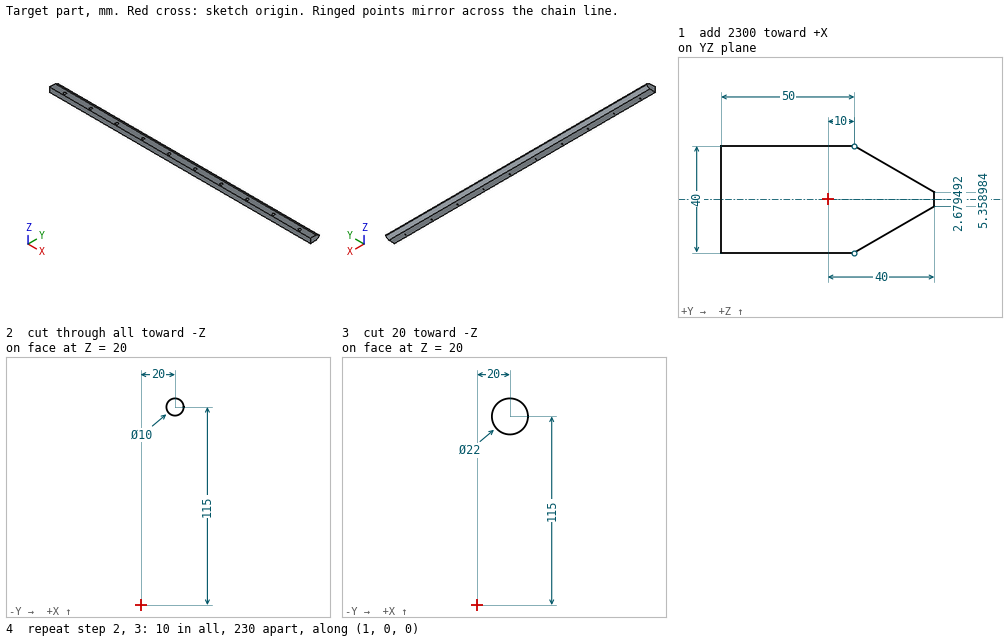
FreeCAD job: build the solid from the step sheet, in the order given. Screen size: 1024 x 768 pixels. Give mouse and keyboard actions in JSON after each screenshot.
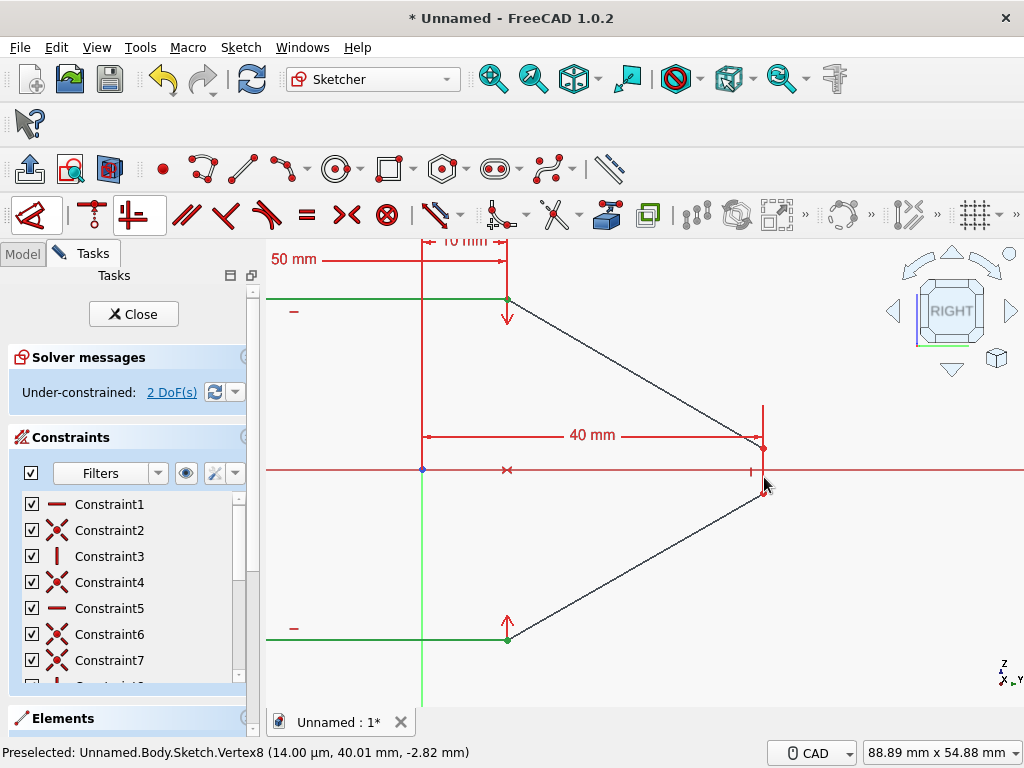
{"action": "left_click", "coordinate": [763, 476]}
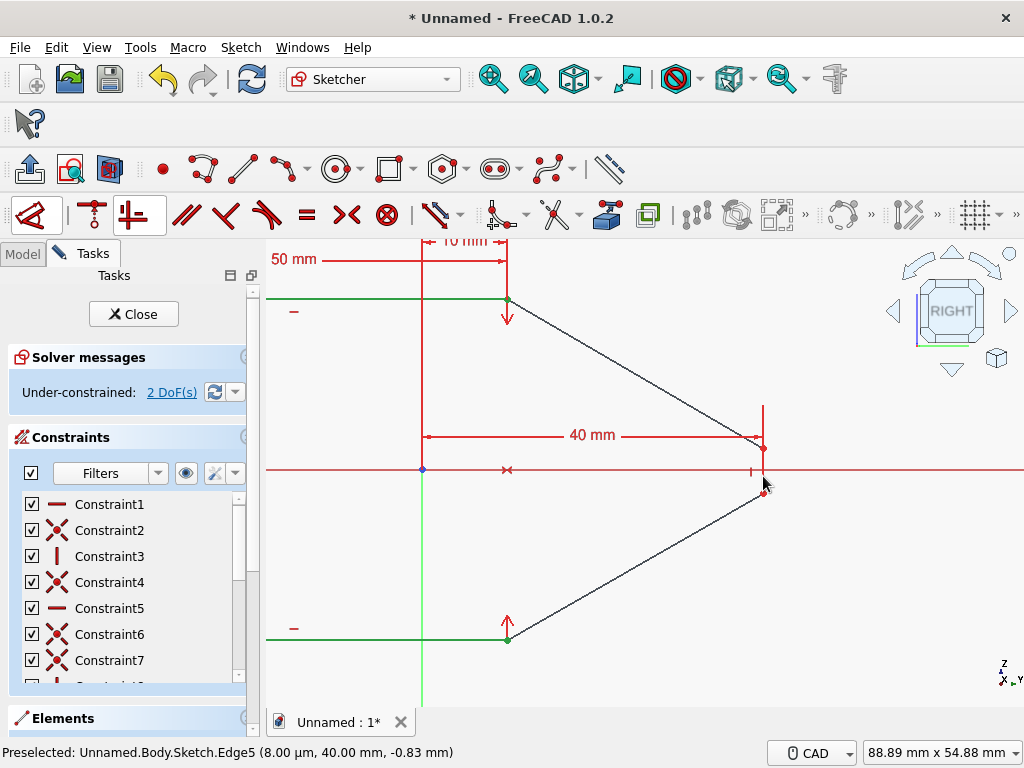
{"action": "key", "text": "i"}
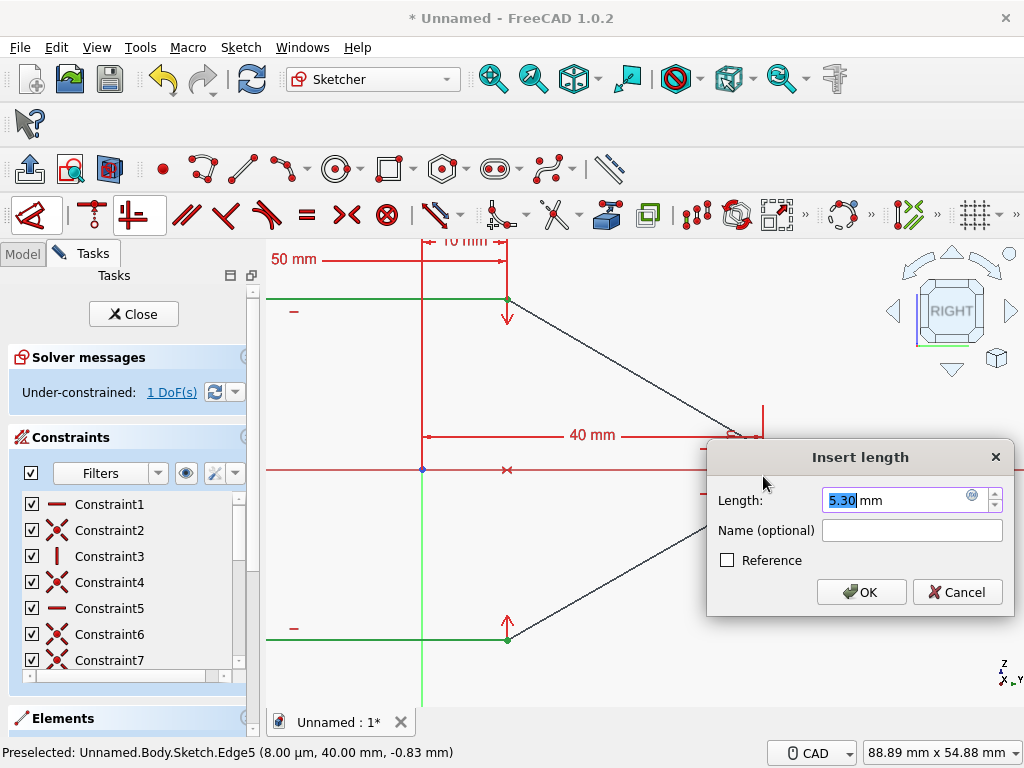
{"action": "type", "text": "5.358984"}
{"action": "key", "text": "Return"}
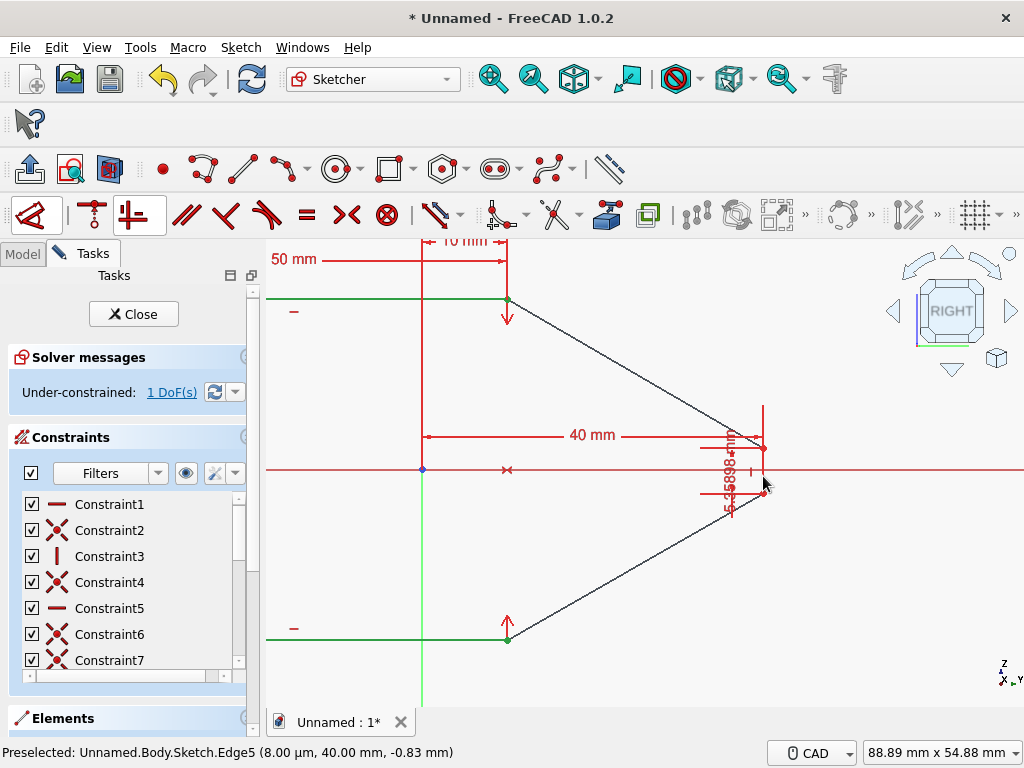
{"action": "scroll", "coordinate": [763, 494], "scroll_direction": "up", "scroll_amount": 3}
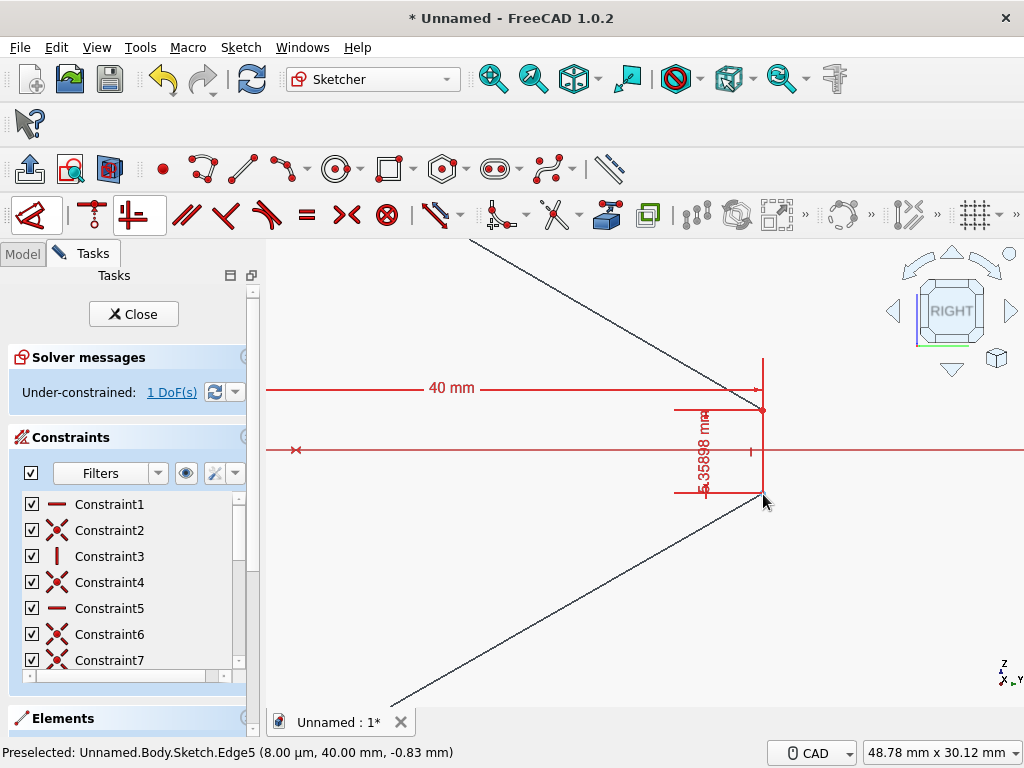
{"action": "left_click", "coordinate": [763, 493]}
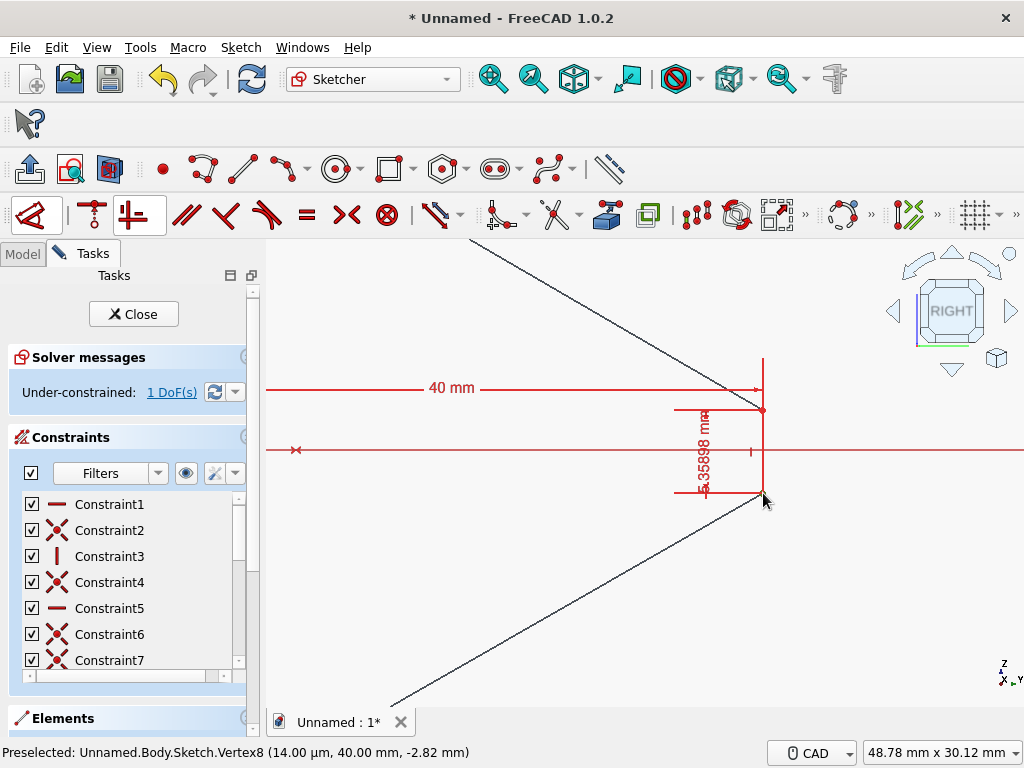
{"action": "key", "text": "i"}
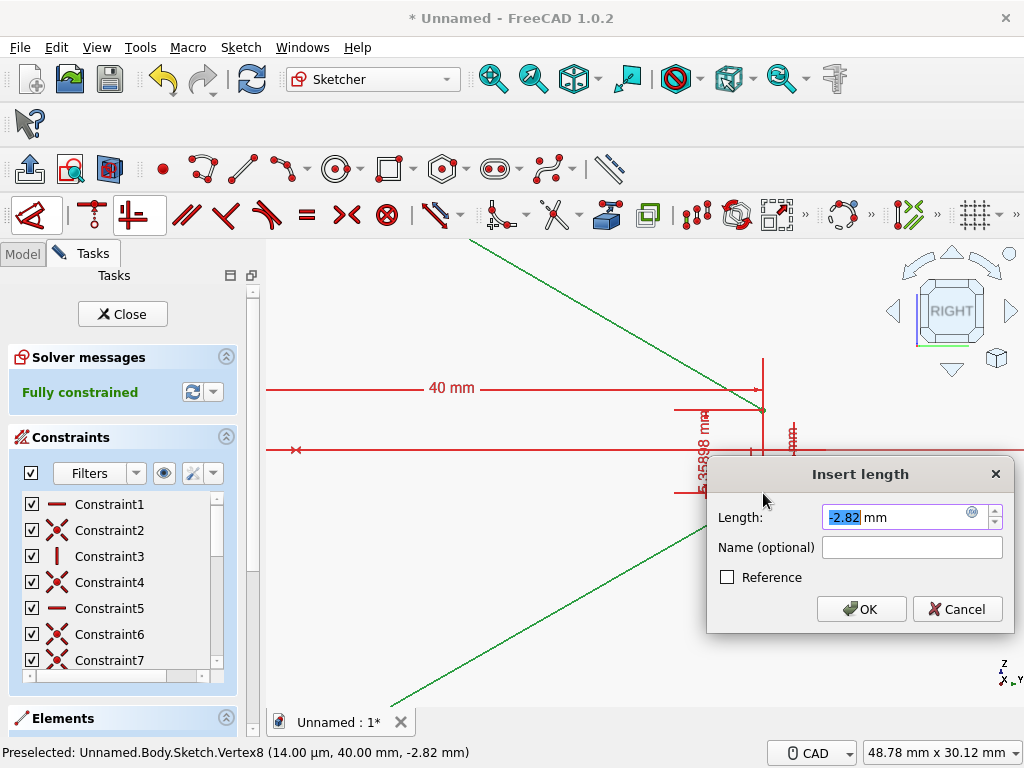
{"action": "type", "text": "-2.679492"}
{"action": "key", "text": "Return"}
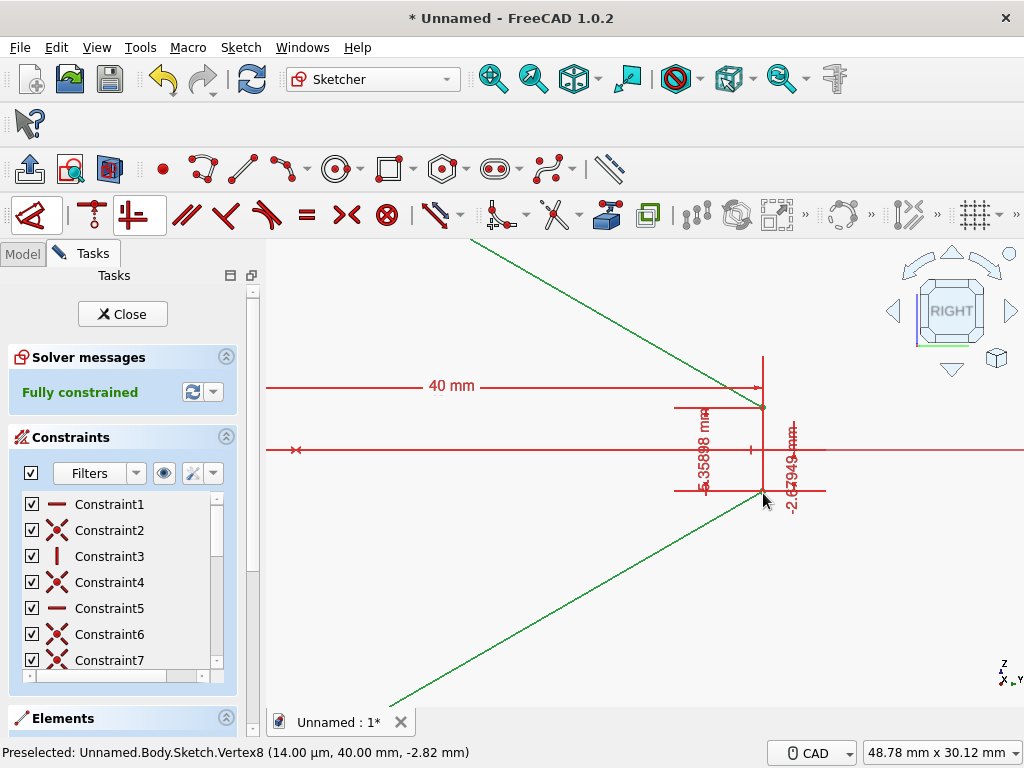
{"action": "left_click", "coordinate": [123, 314]}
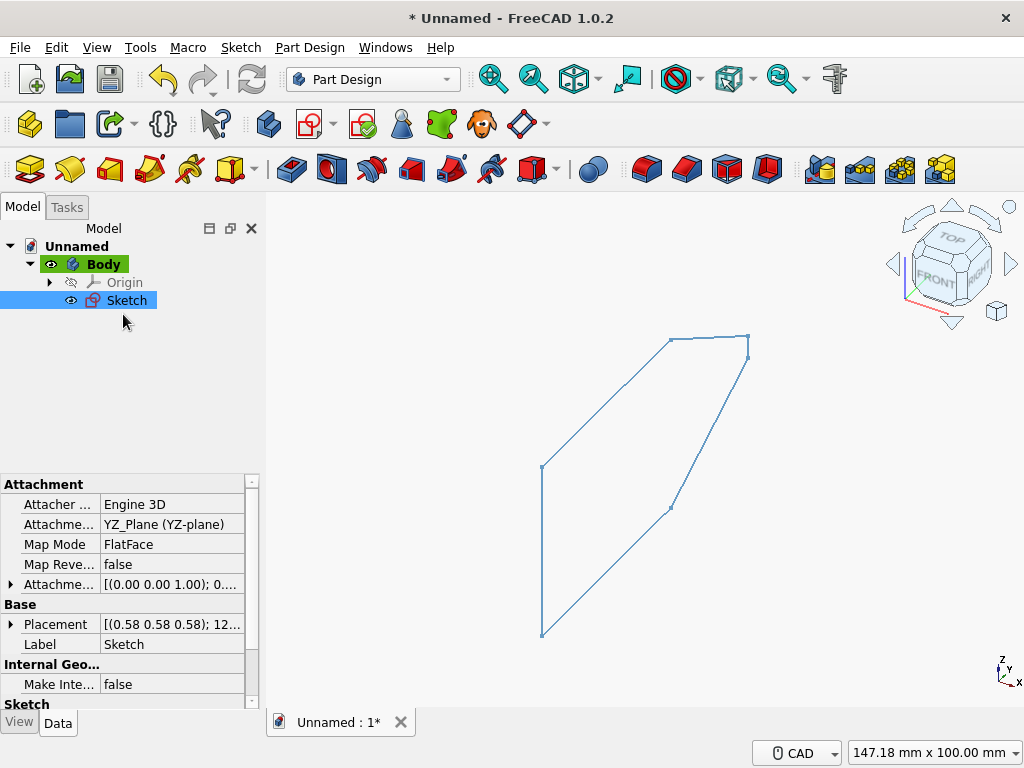
{"action": "left_click", "coordinate": [30, 170]}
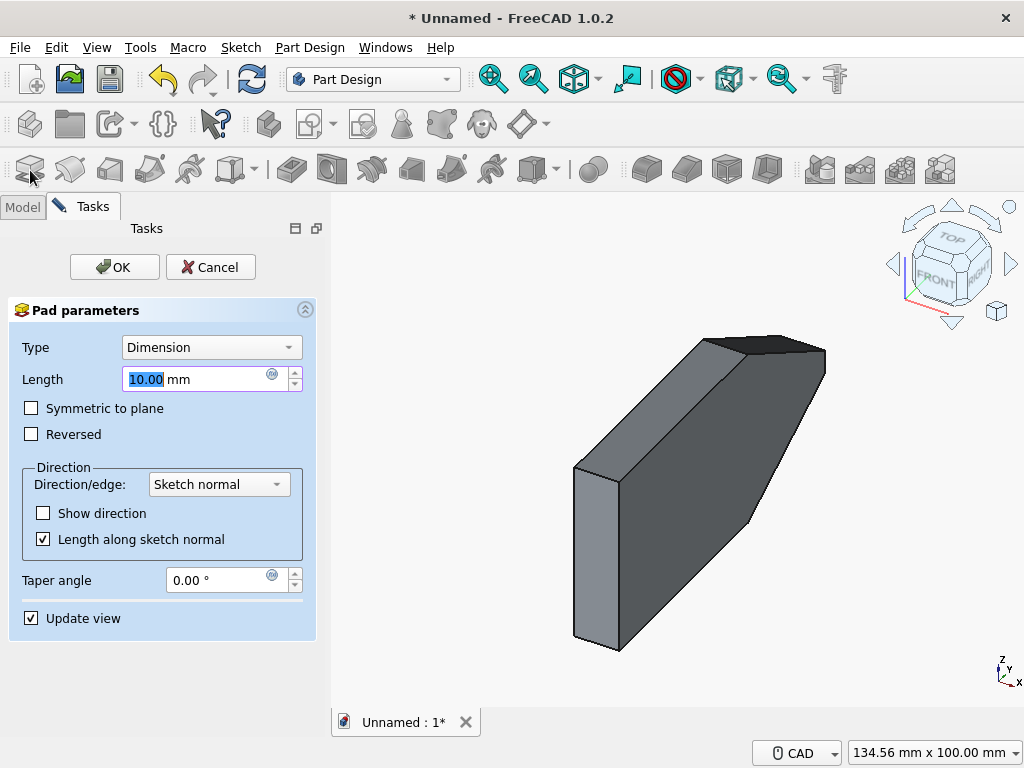
{"action": "type", "text": "2300"}
{"action": "key", "text": "Tab"}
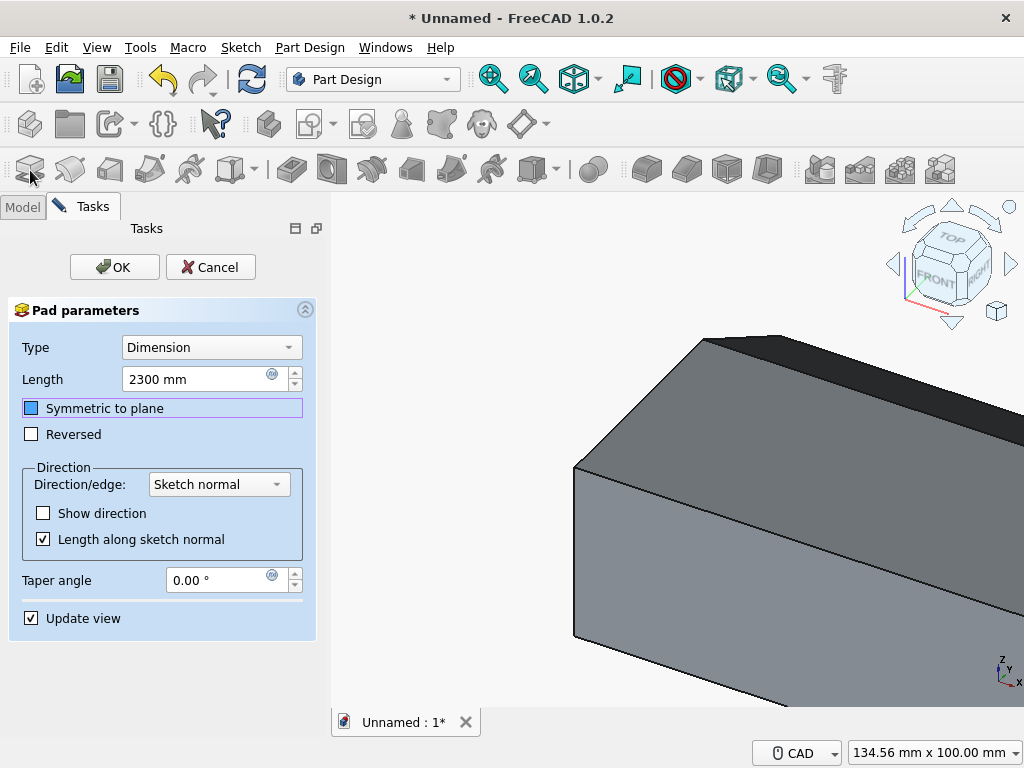
{"action": "left_click", "coordinate": [115, 267]}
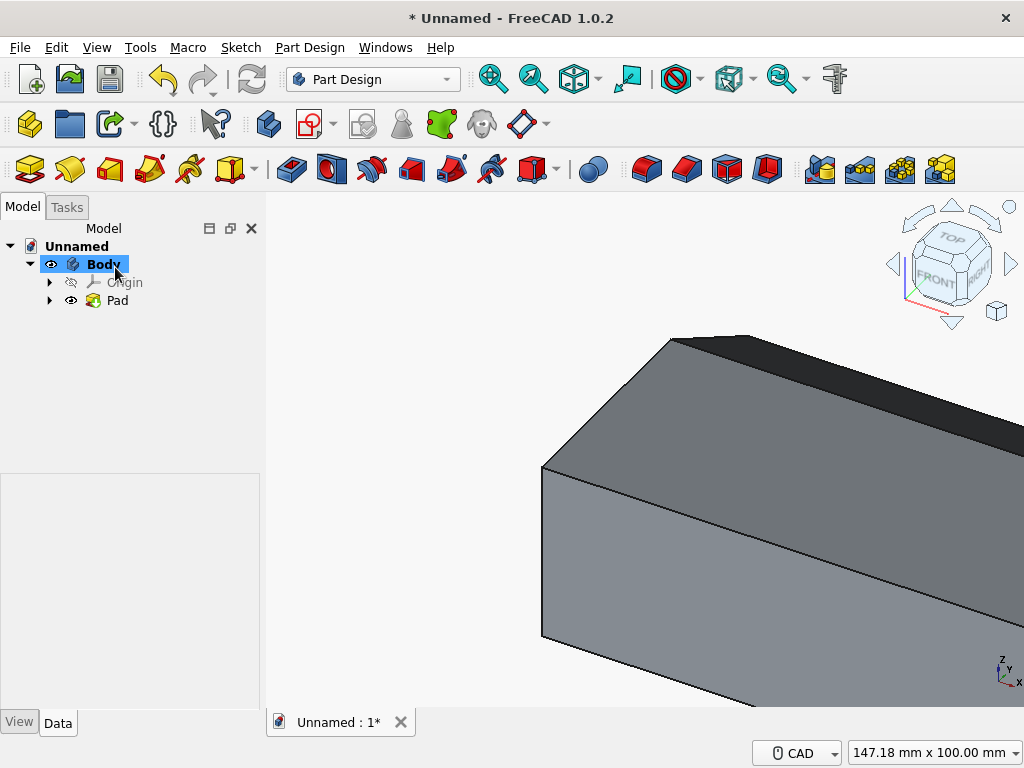
{"action": "left_click", "coordinate": [494, 80]}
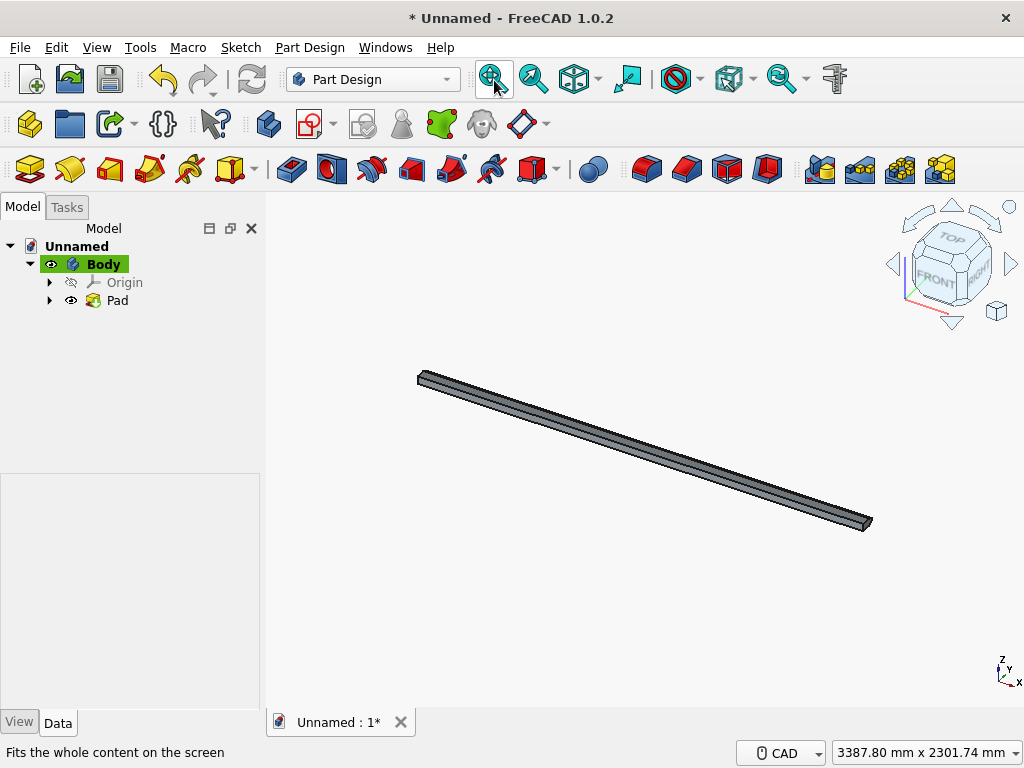
{"action": "scroll", "coordinate": [643, 447], "scroll_direction": "up", "scroll_amount": 4}